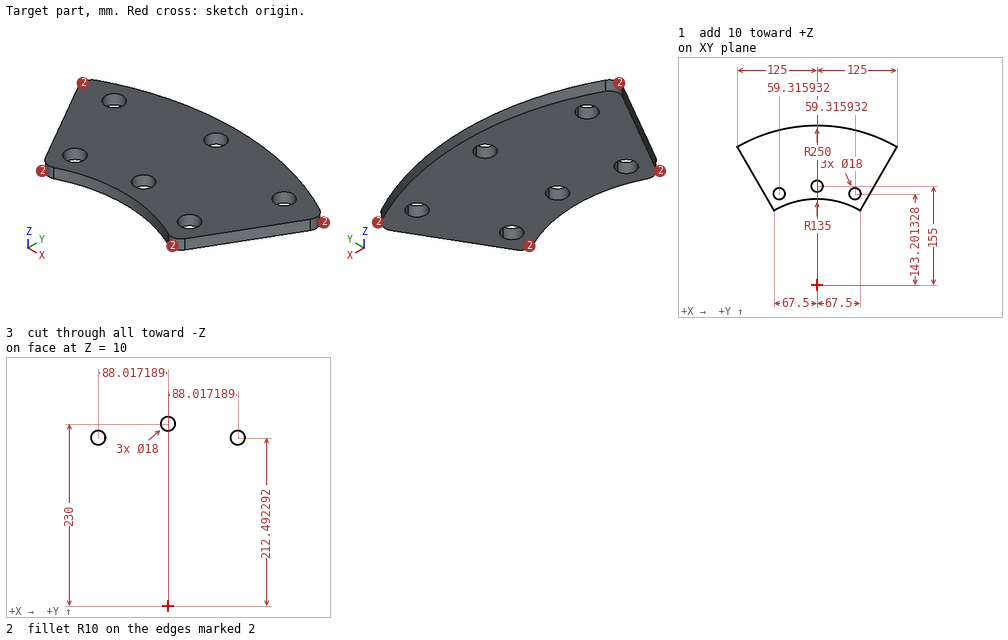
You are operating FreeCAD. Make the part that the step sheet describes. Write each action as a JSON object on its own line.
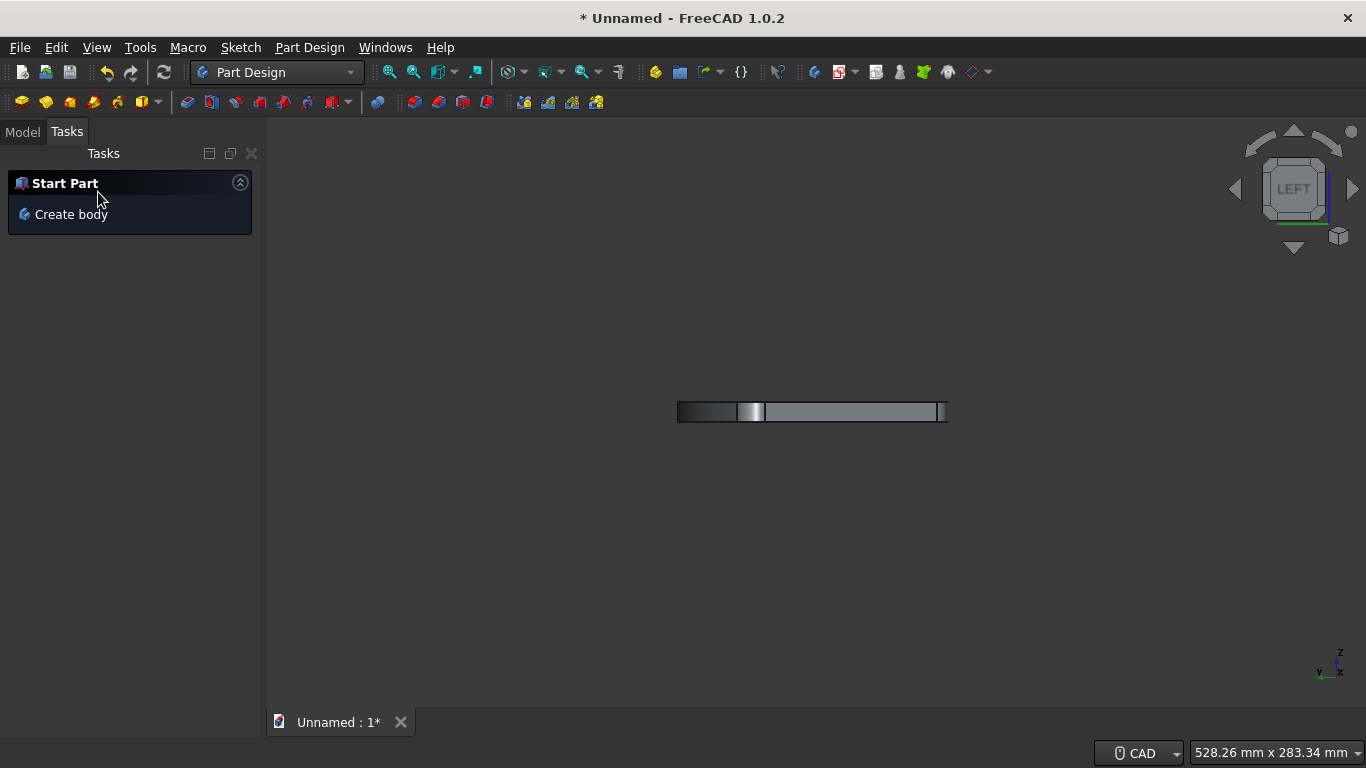
{"action": "left_click", "coordinate": [390, 72]}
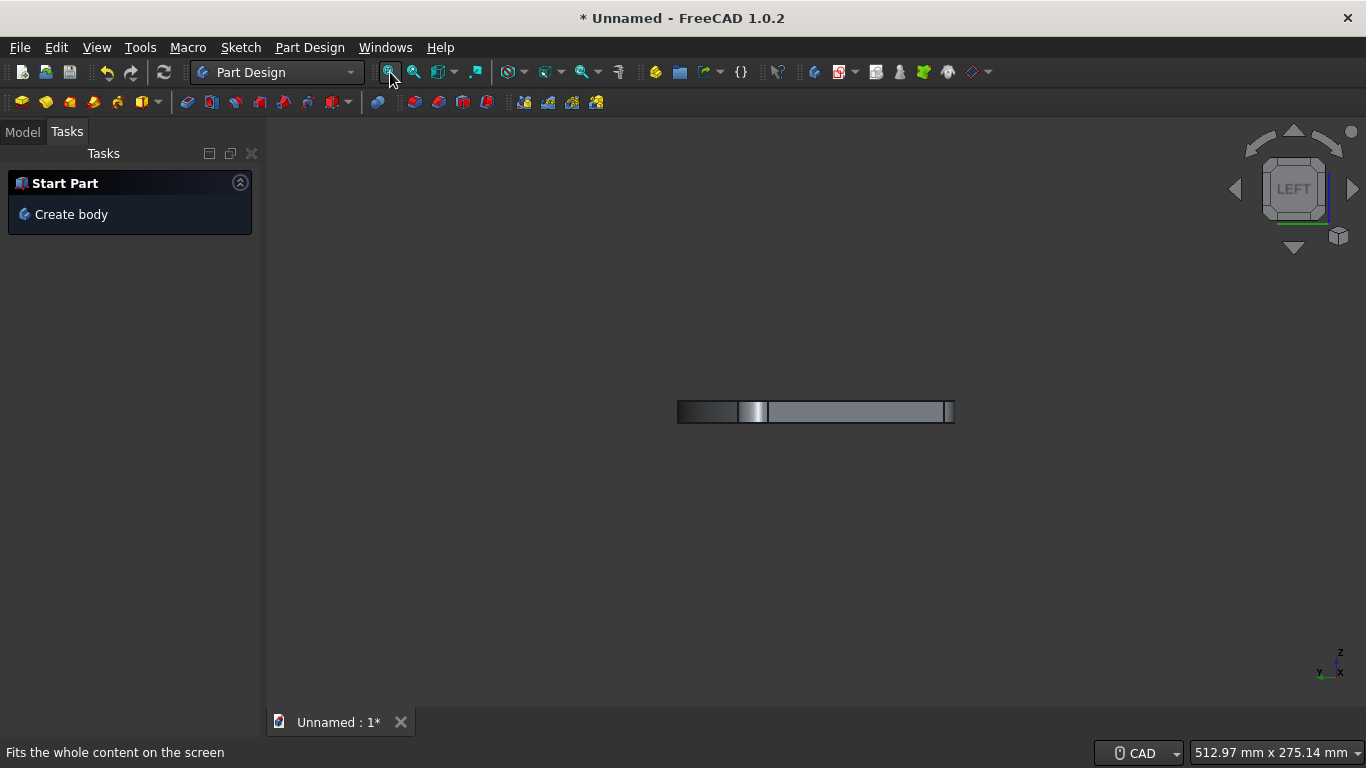
{"action": "key", "text": "0"}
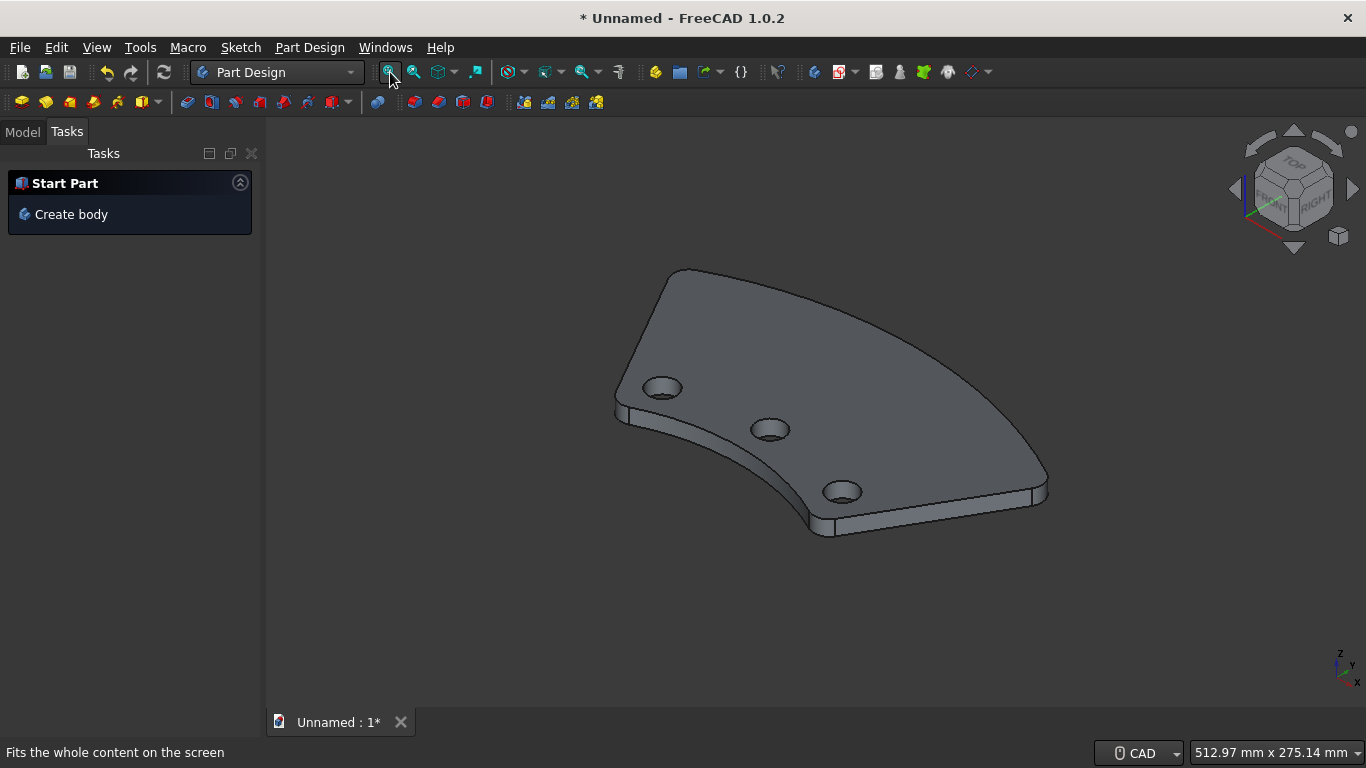
{"action": "left_click", "coordinate": [897, 416]}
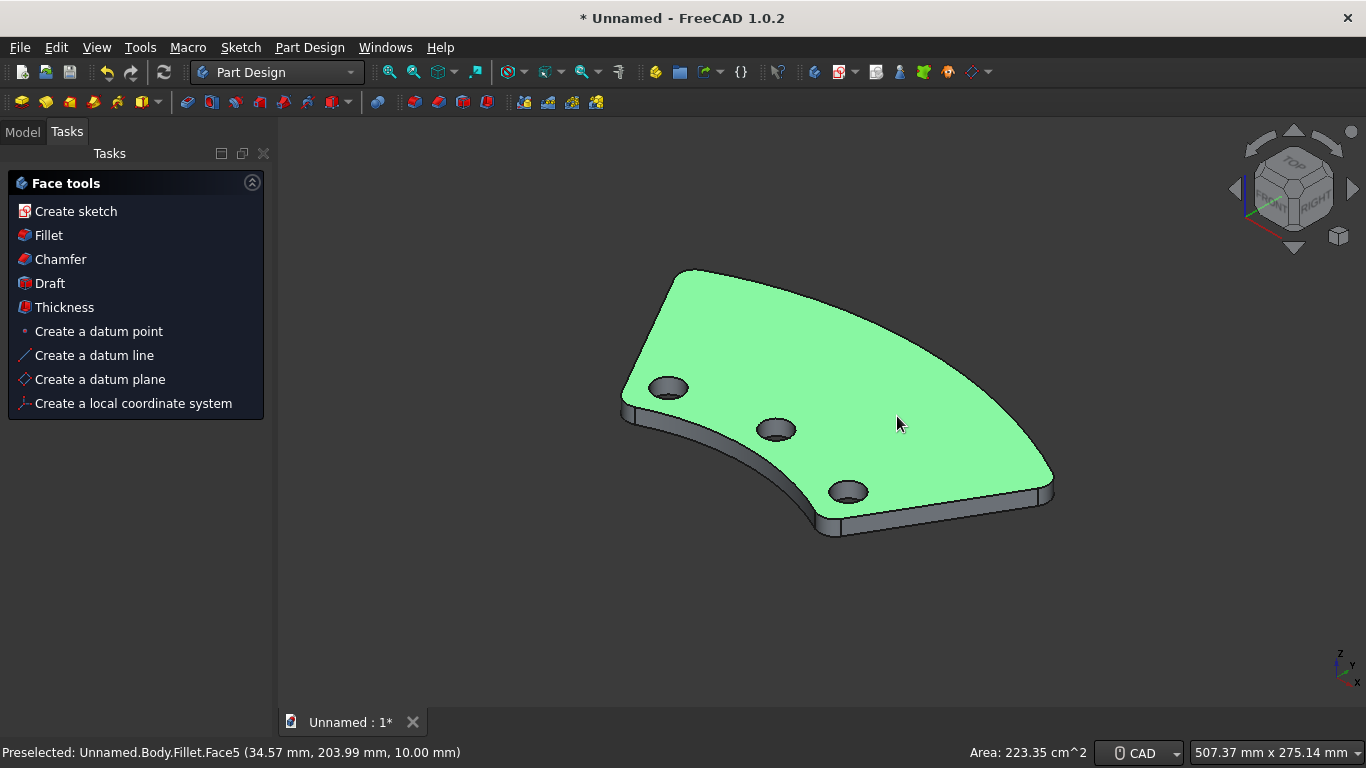
{"action": "left_click", "coordinate": [840, 72]}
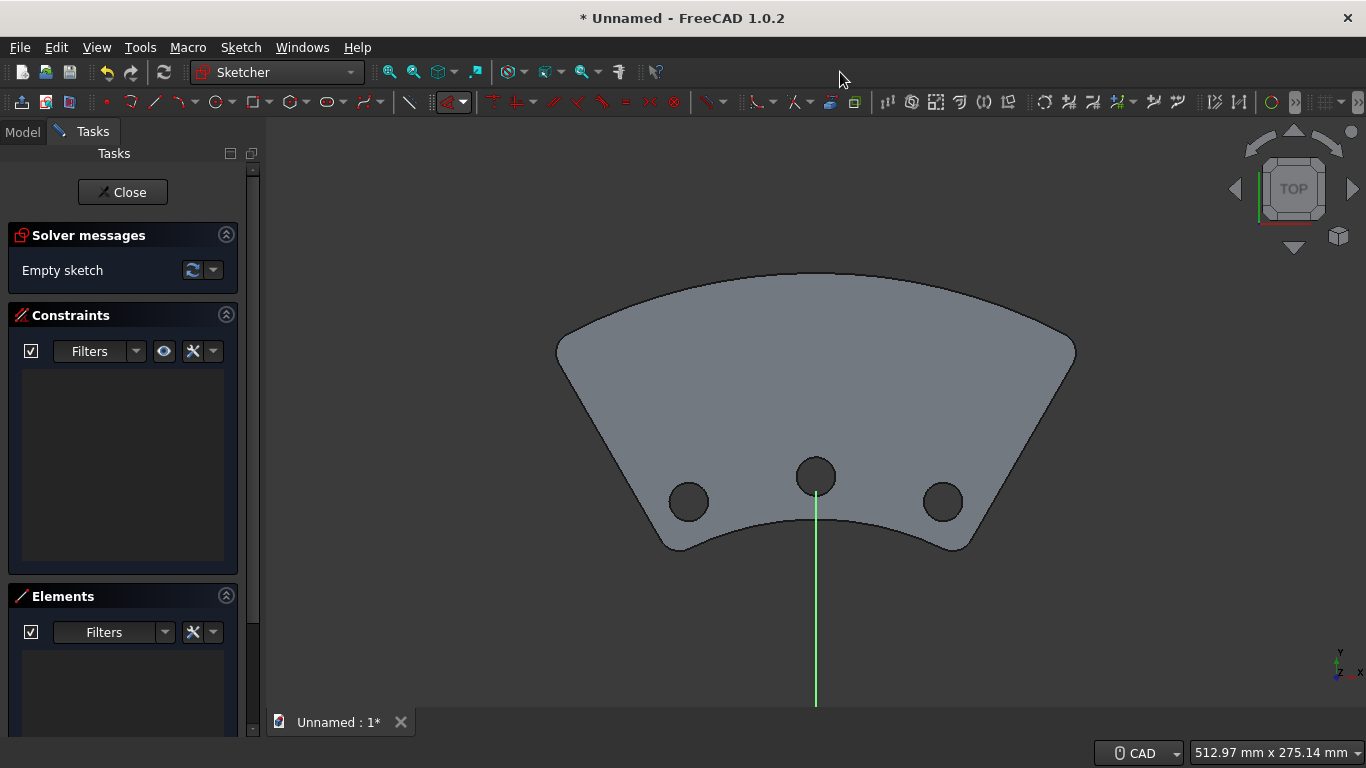
{"action": "scroll", "coordinate": [608, 145], "scroll_direction": "down", "scroll_amount": 2}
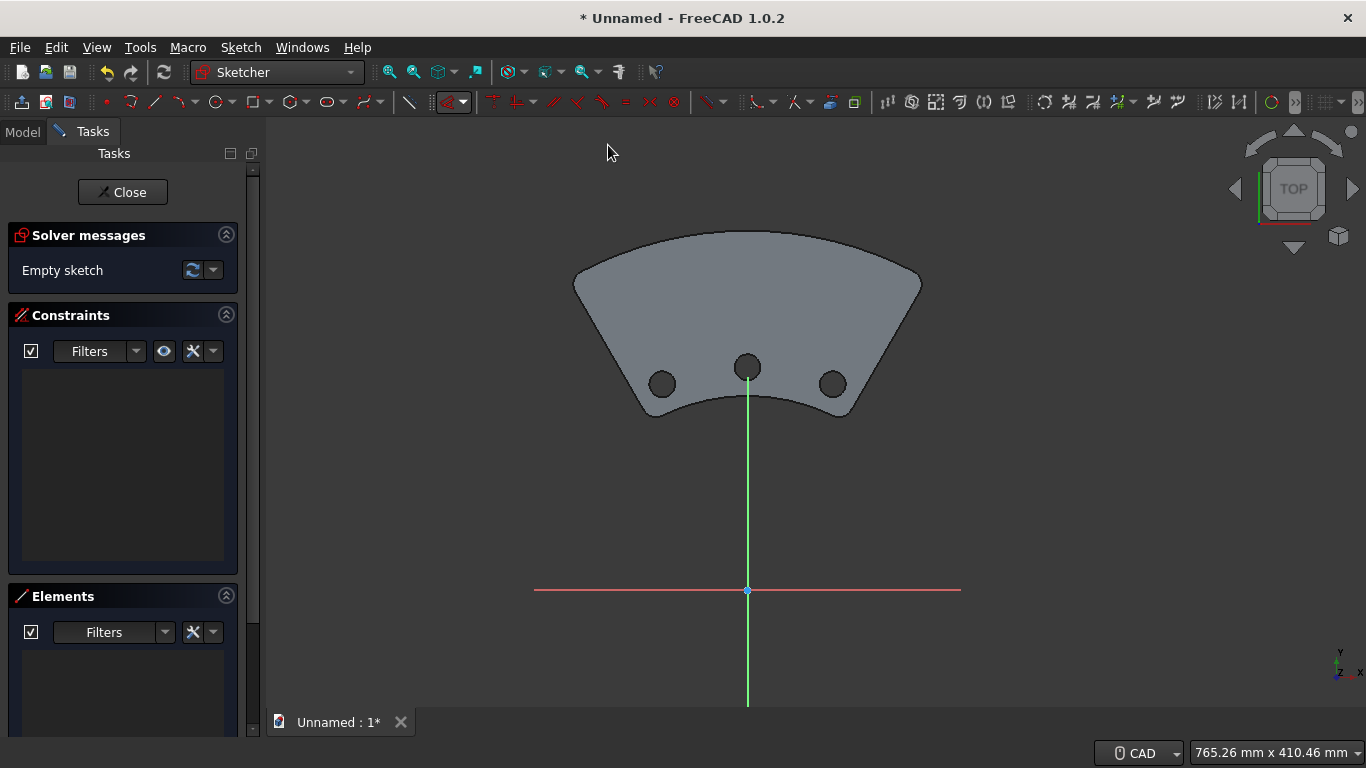
{"action": "left_click", "coordinate": [216, 102]}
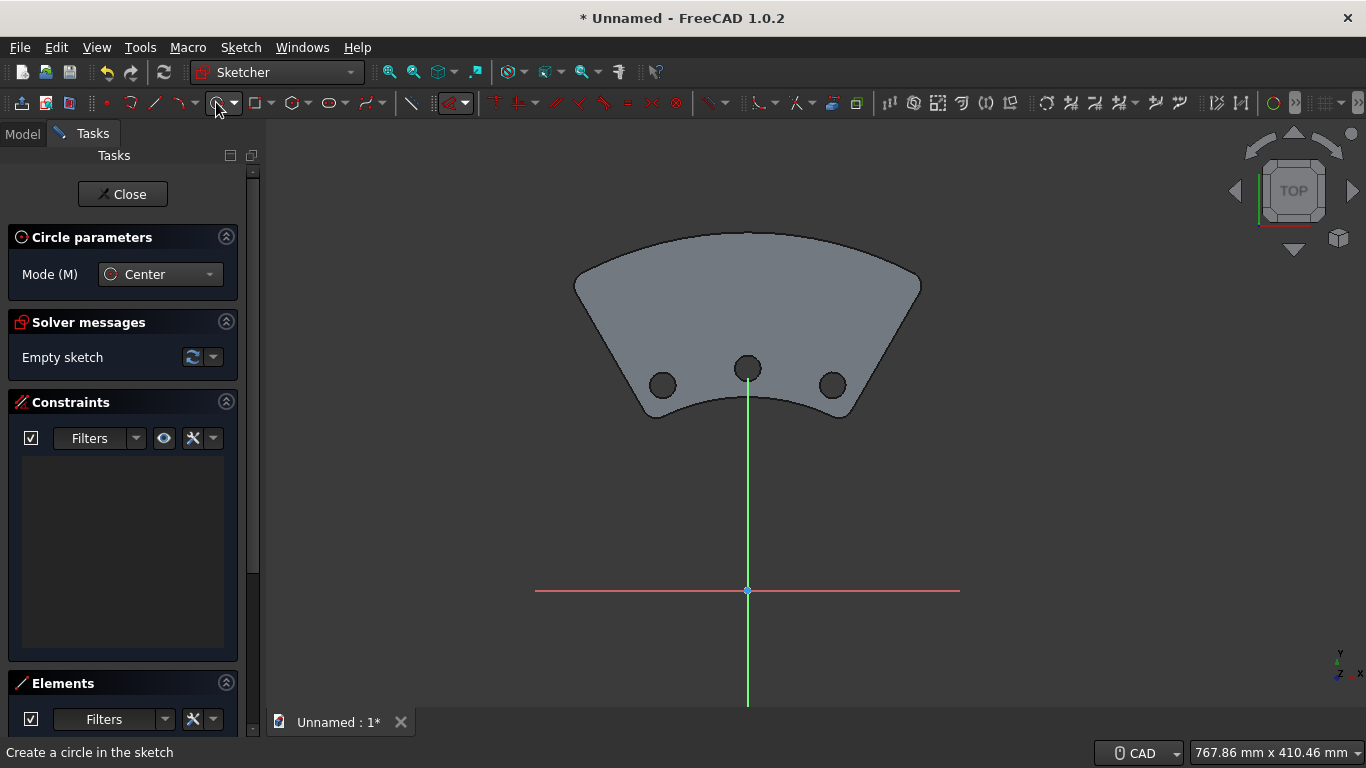
{"action": "scroll", "coordinate": [748, 261], "scroll_direction": "up", "scroll_amount": 3}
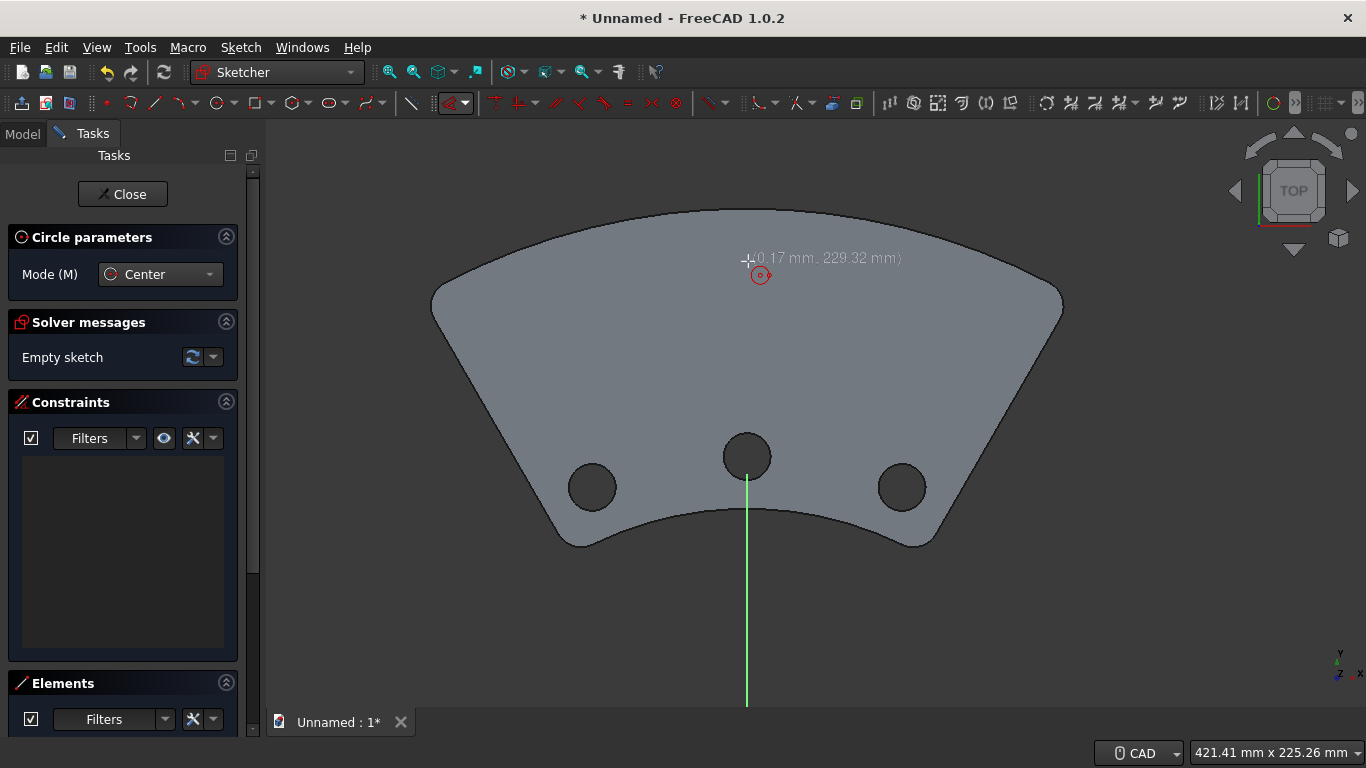
{"action": "left_click", "coordinate": [747, 261]}
{"action": "mouse_move", "coordinate": [764, 244]}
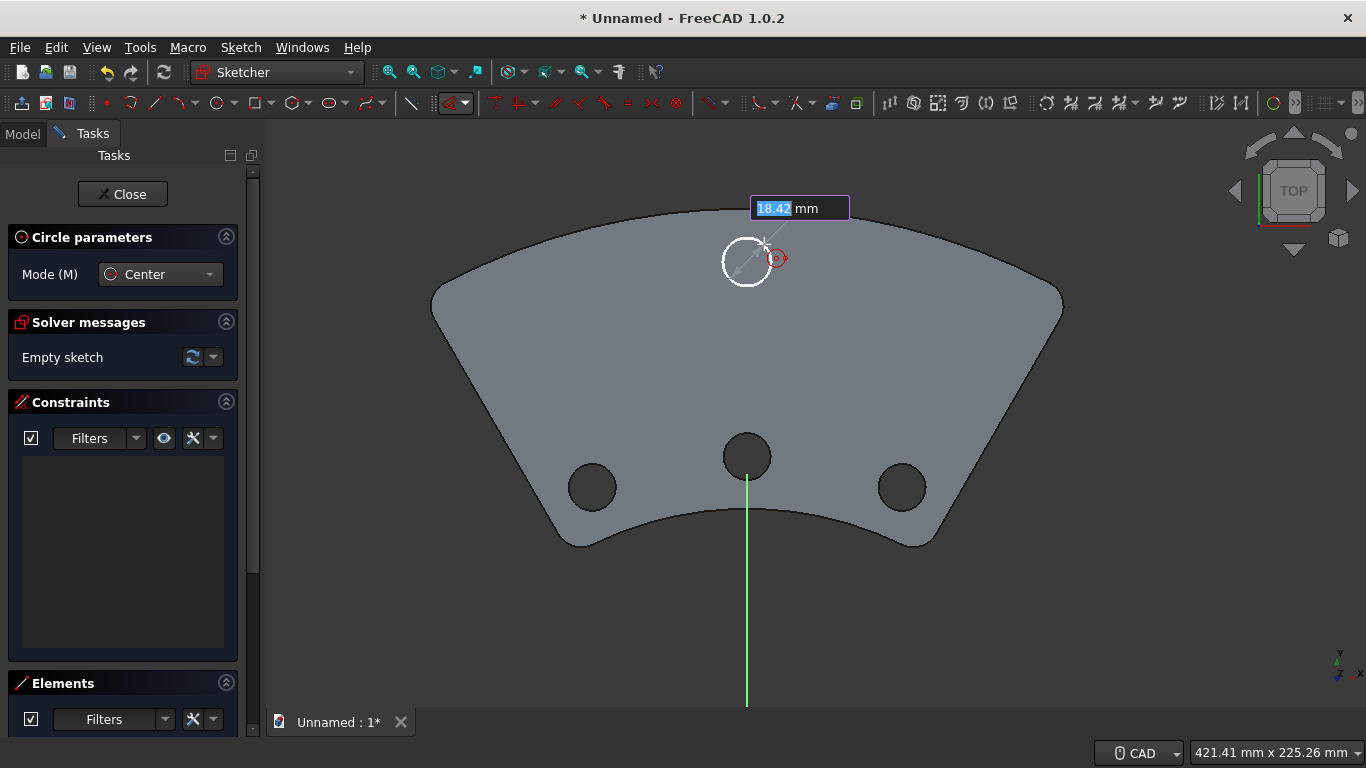
{"action": "type", "text": "18"}
{"action": "key", "text": "Return"}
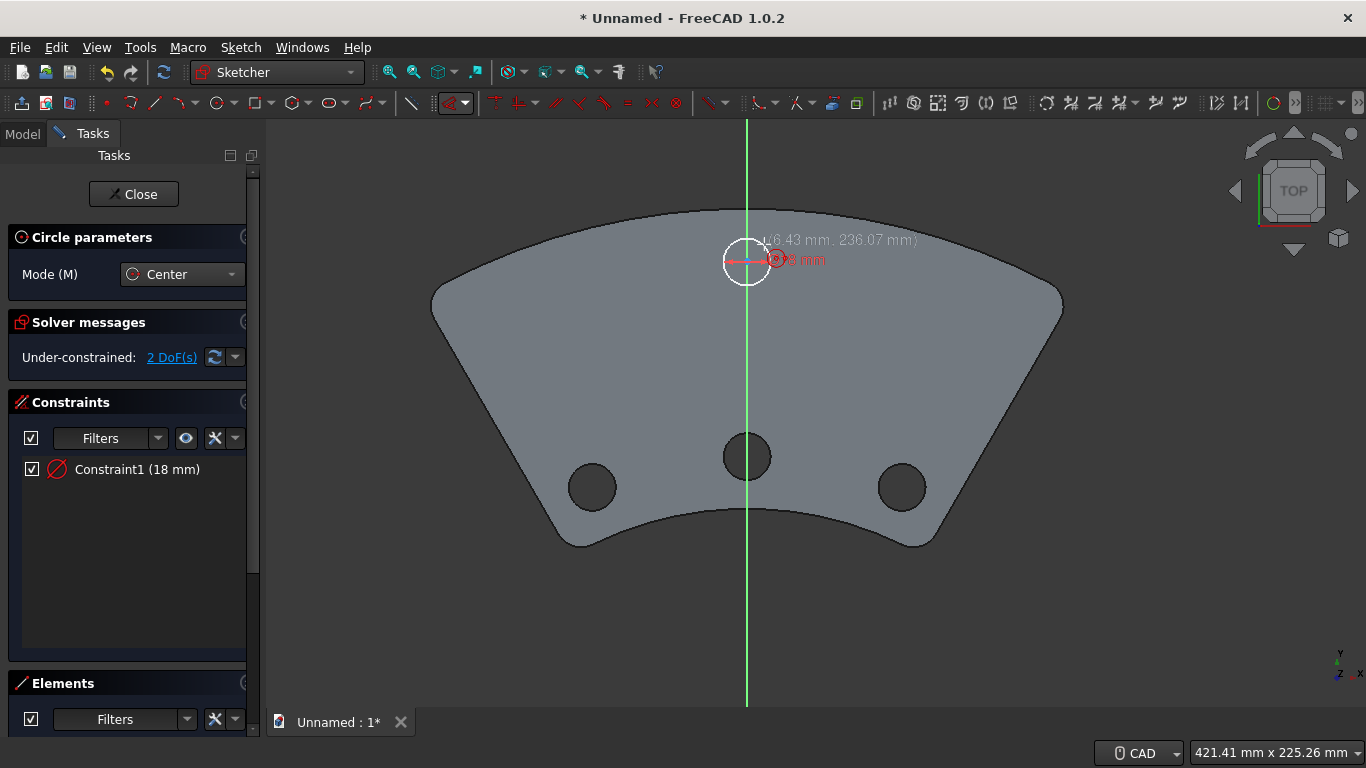
{"action": "left_click", "coordinate": [977, 307]}
{"action": "mouse_move", "coordinate": [994, 290]}